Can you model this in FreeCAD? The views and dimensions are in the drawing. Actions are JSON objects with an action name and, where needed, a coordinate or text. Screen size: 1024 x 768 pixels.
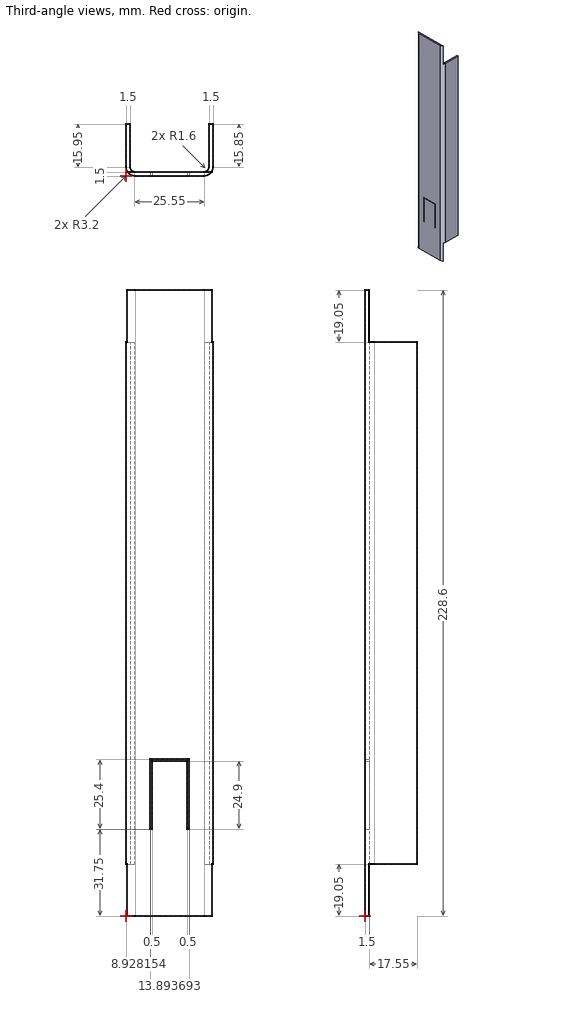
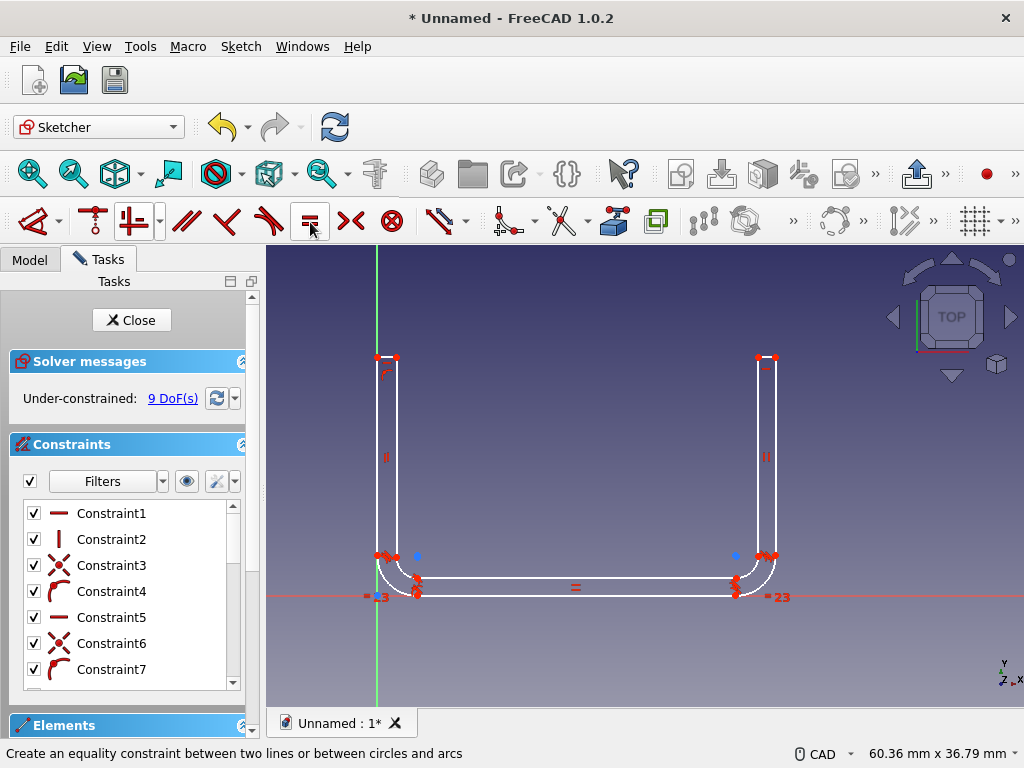
{"action": "scroll", "coordinate": [399, 567], "scroll_direction": "up", "scroll_amount": 2}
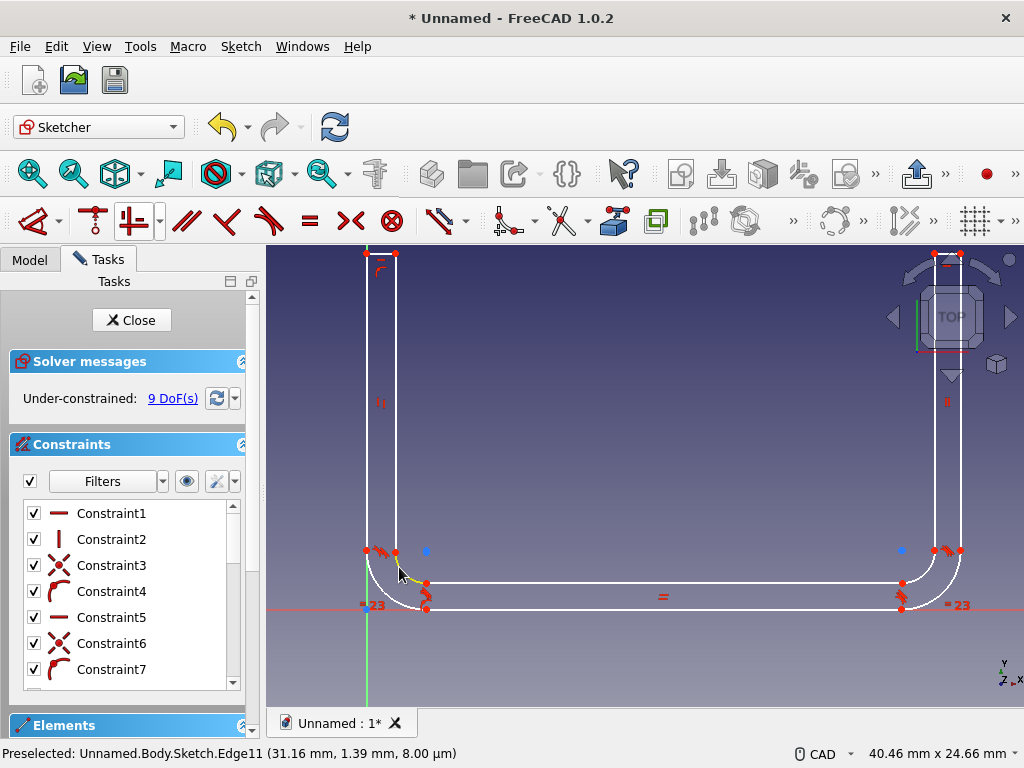
{"action": "left_click", "coordinate": [399, 566]}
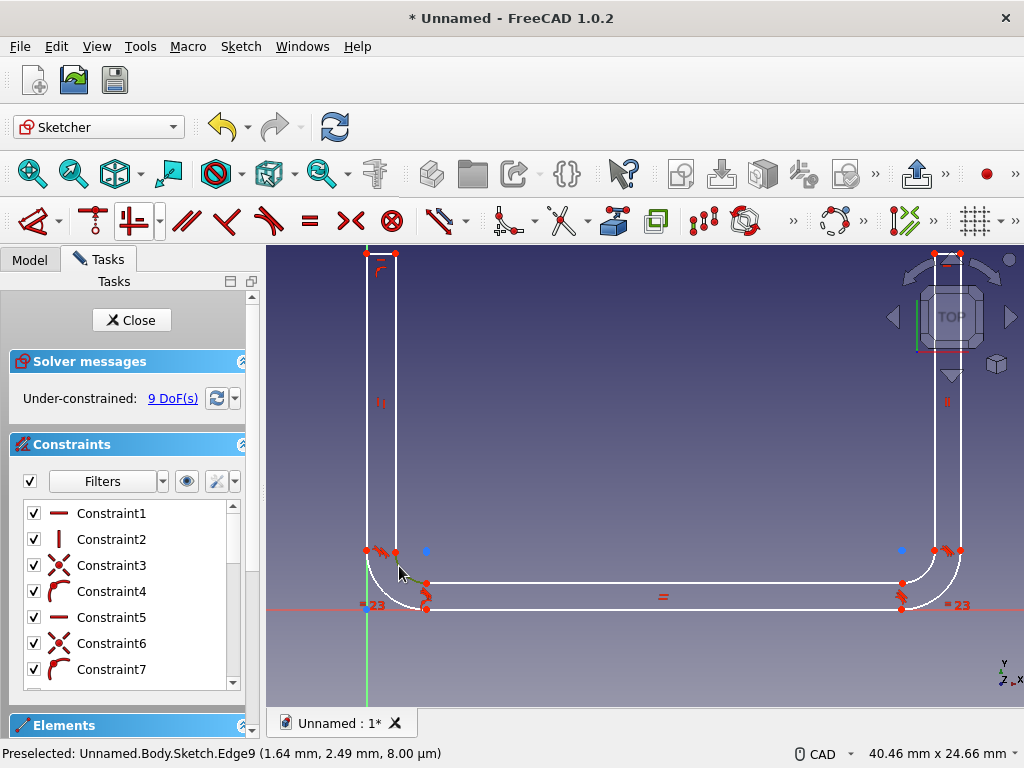
{"action": "scroll", "coordinate": [398, 567], "scroll_direction": "down", "scroll_amount": 2}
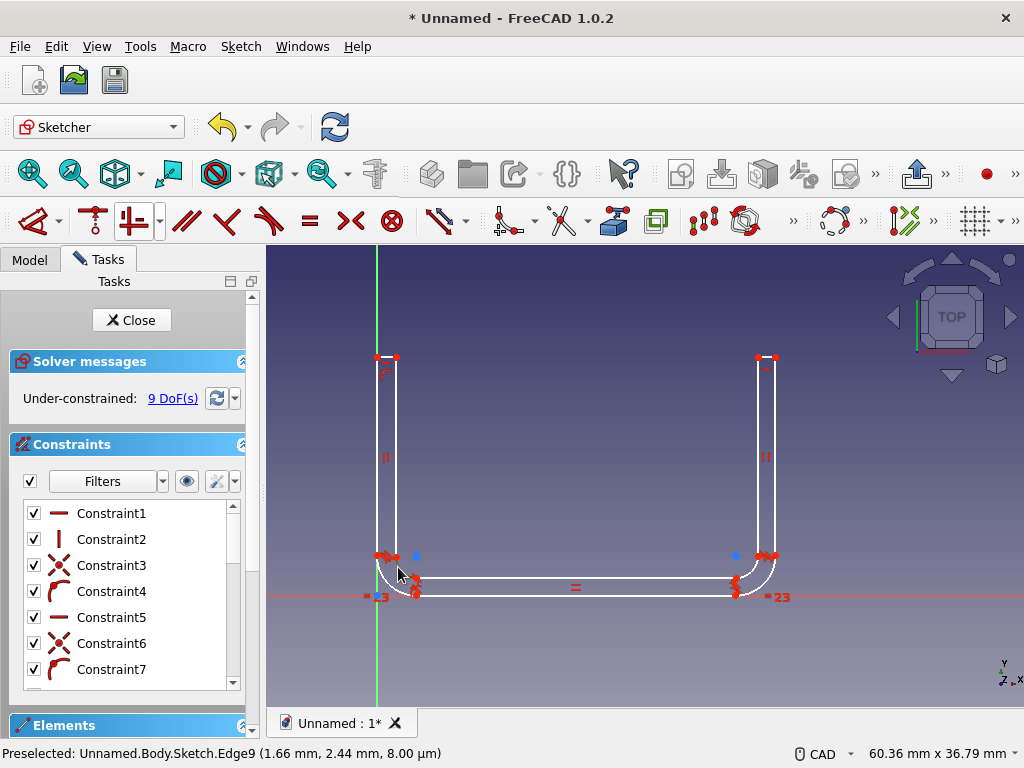
{"action": "scroll", "coordinate": [746, 576], "scroll_direction": "up", "scroll_amount": 2}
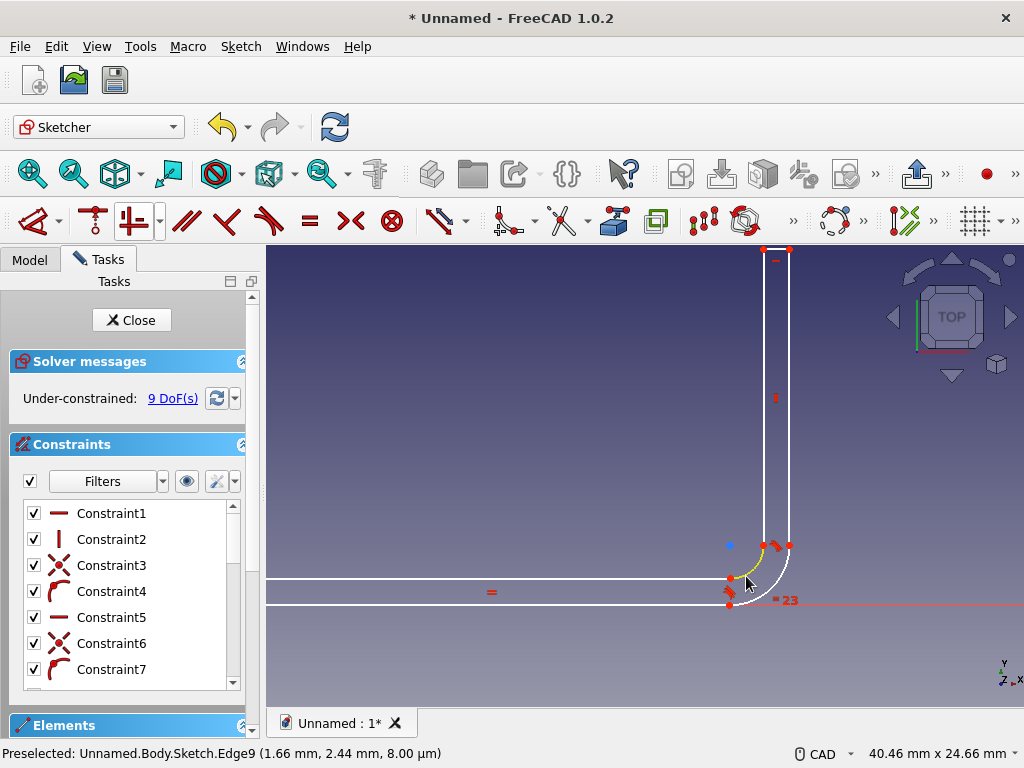
{"action": "left_click", "coordinate": [746, 575]}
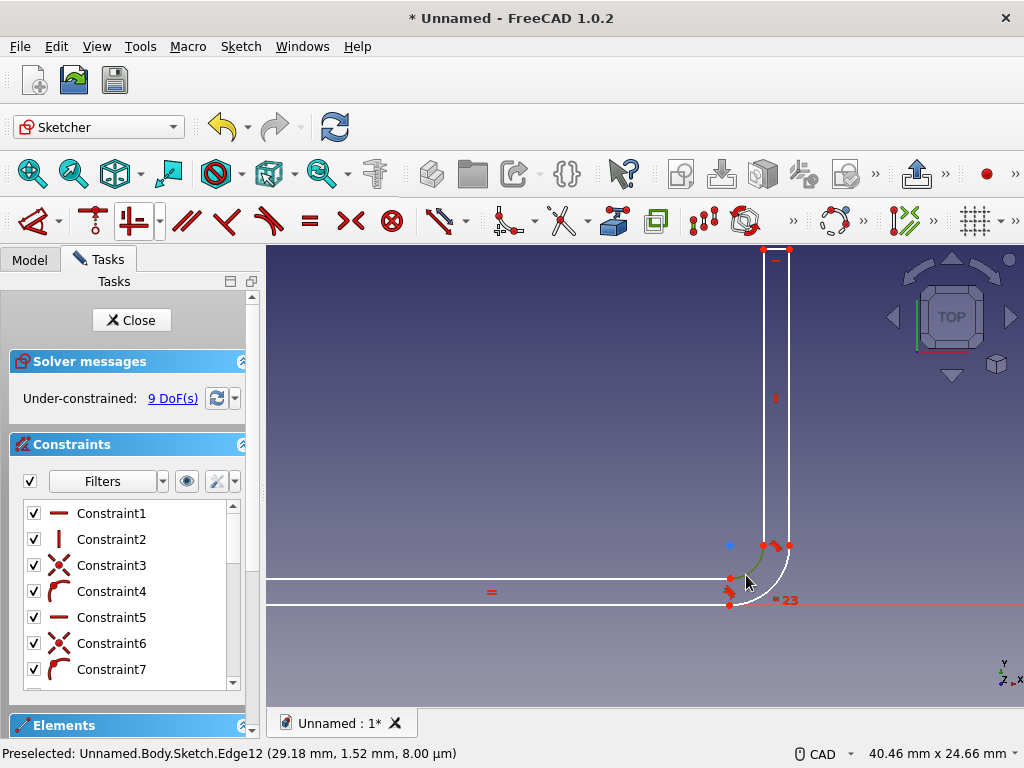
{"action": "left_click", "coordinate": [310, 222]}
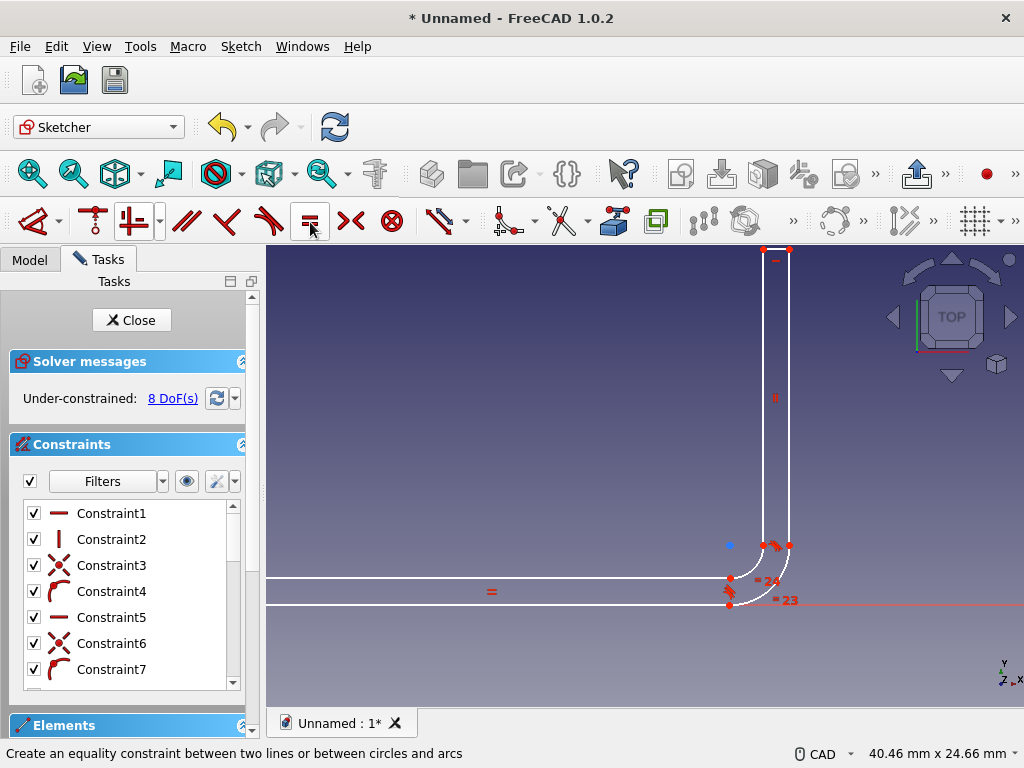
{"action": "scroll", "coordinate": [747, 576], "scroll_direction": "down", "scroll_amount": 2}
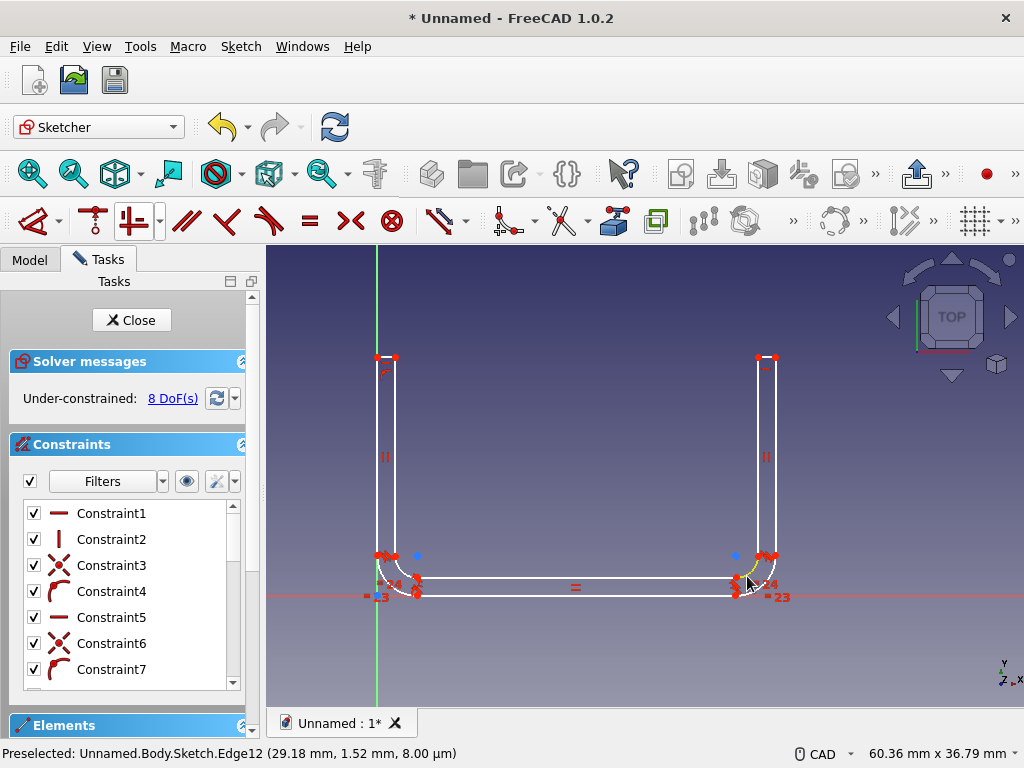
{"action": "scroll", "coordinate": [398, 566], "scroll_direction": "up", "scroll_amount": 4}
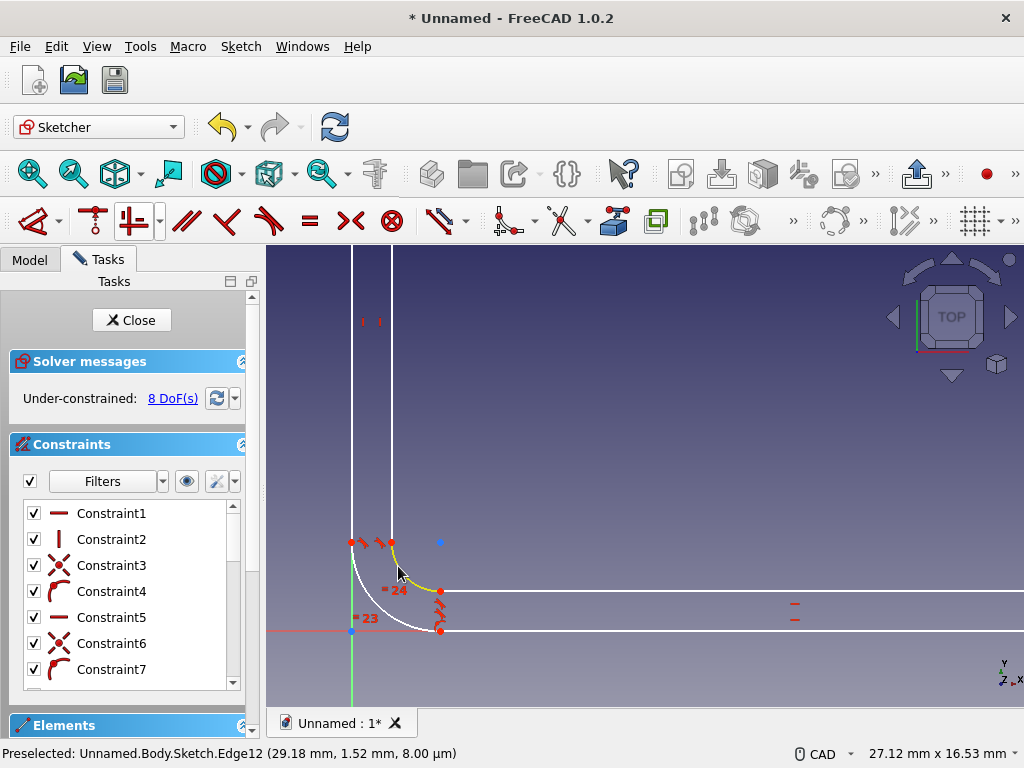
{"action": "left_click", "coordinate": [397, 565]}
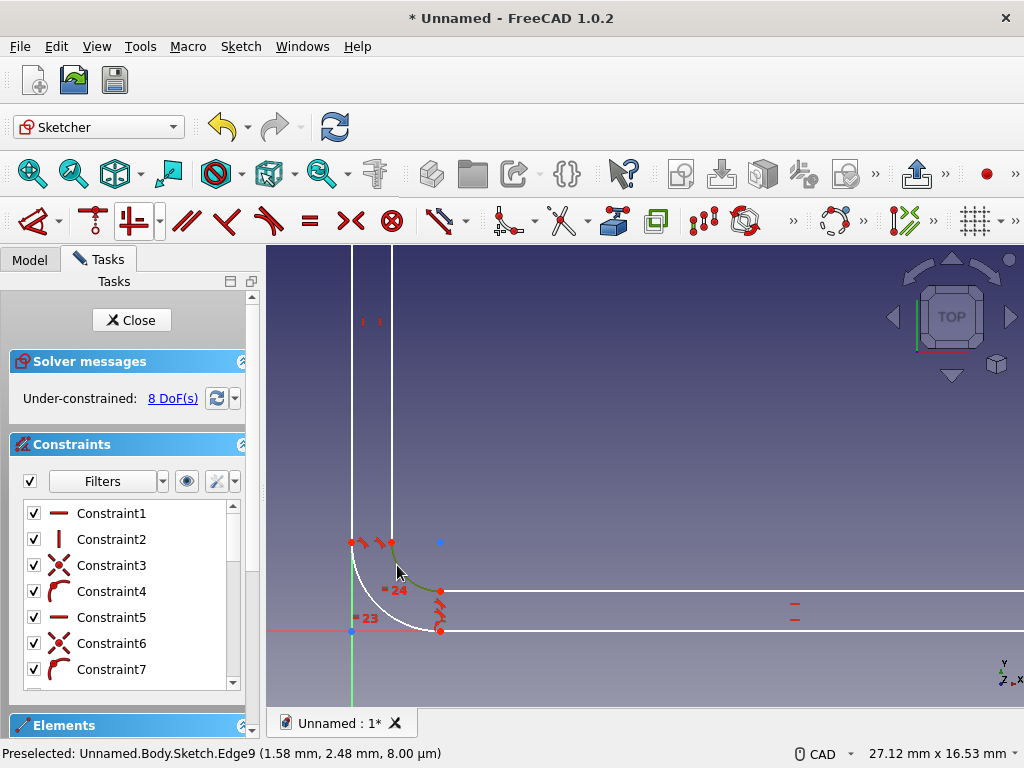
{"action": "key", "text": "k r"}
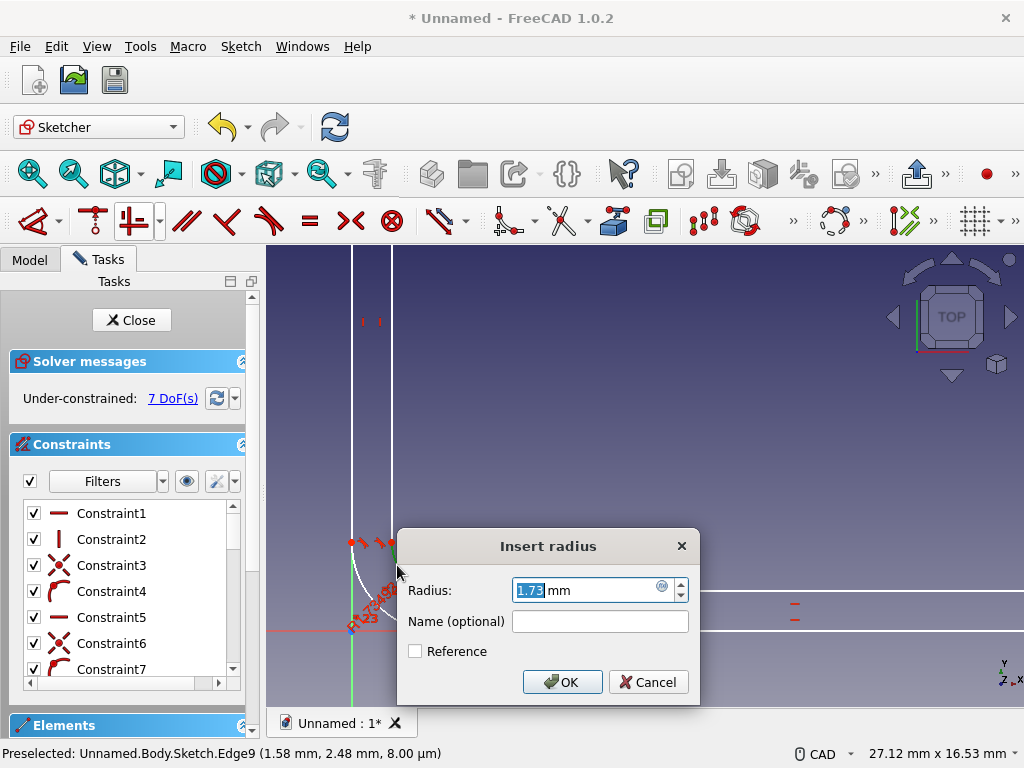
{"action": "type", "text": "1.6"}
{"action": "key", "text": "Return"}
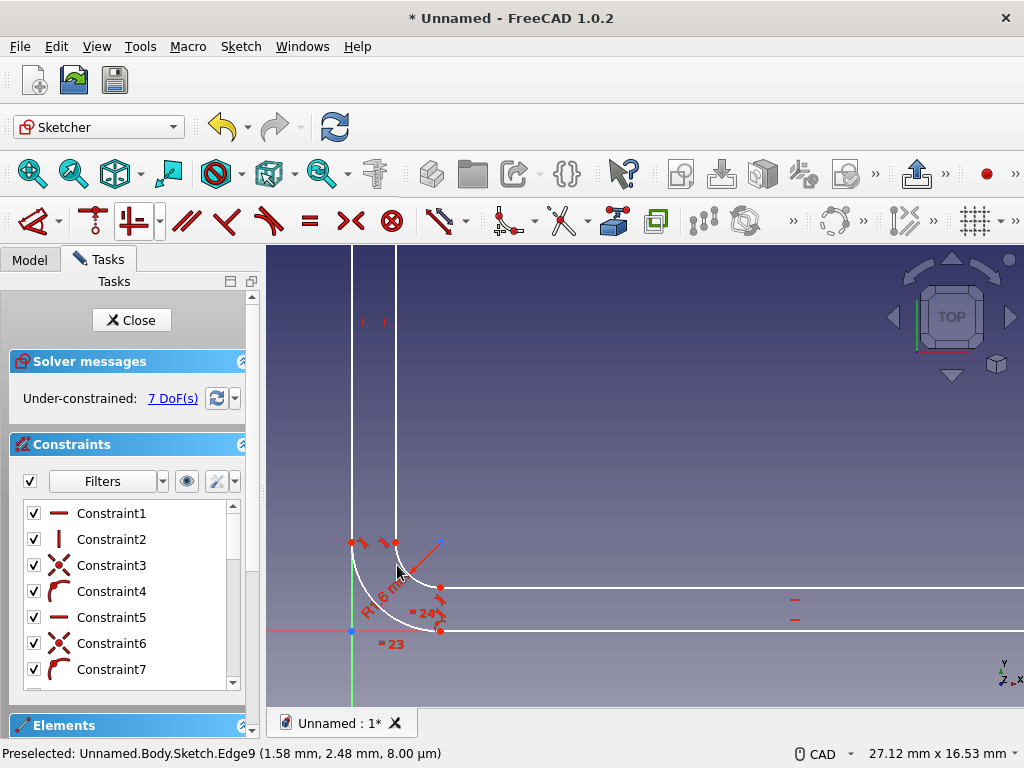
{"action": "scroll", "coordinate": [362, 583], "scroll_direction": "up", "scroll_amount": 2}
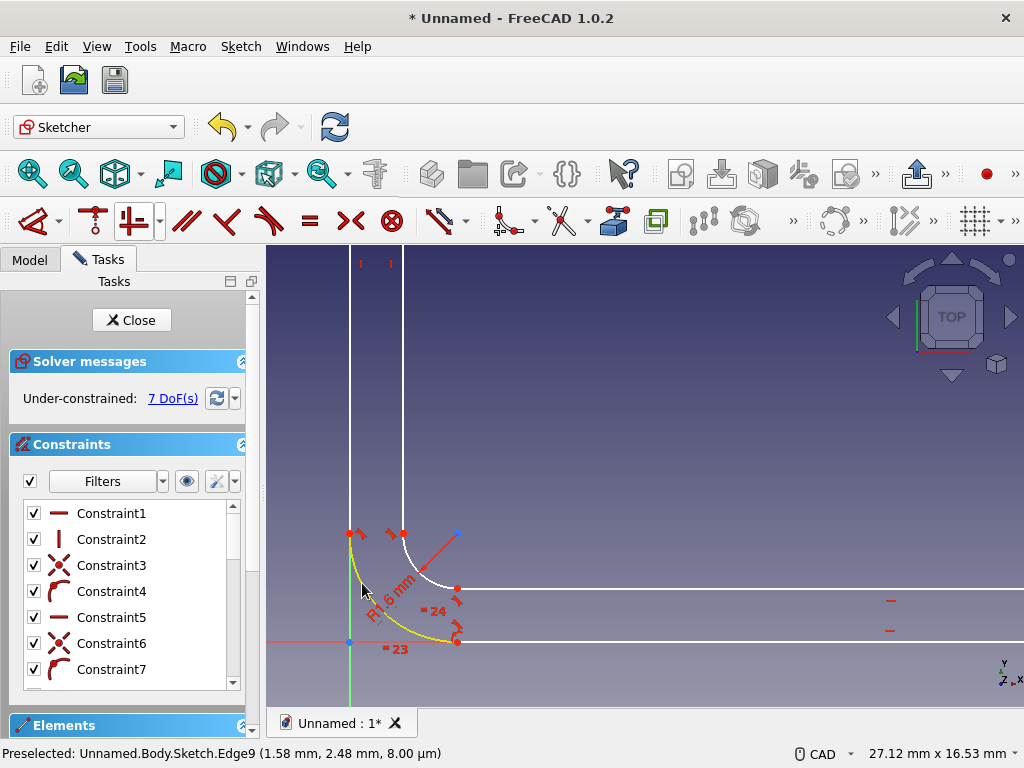
{"action": "left_click", "coordinate": [361, 583]}